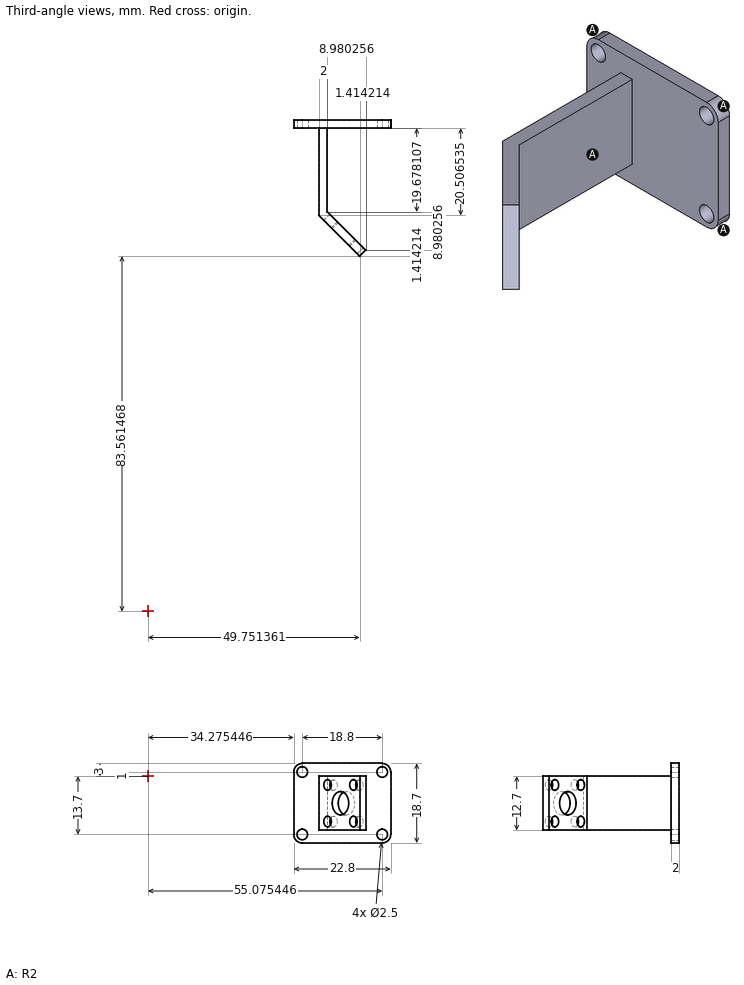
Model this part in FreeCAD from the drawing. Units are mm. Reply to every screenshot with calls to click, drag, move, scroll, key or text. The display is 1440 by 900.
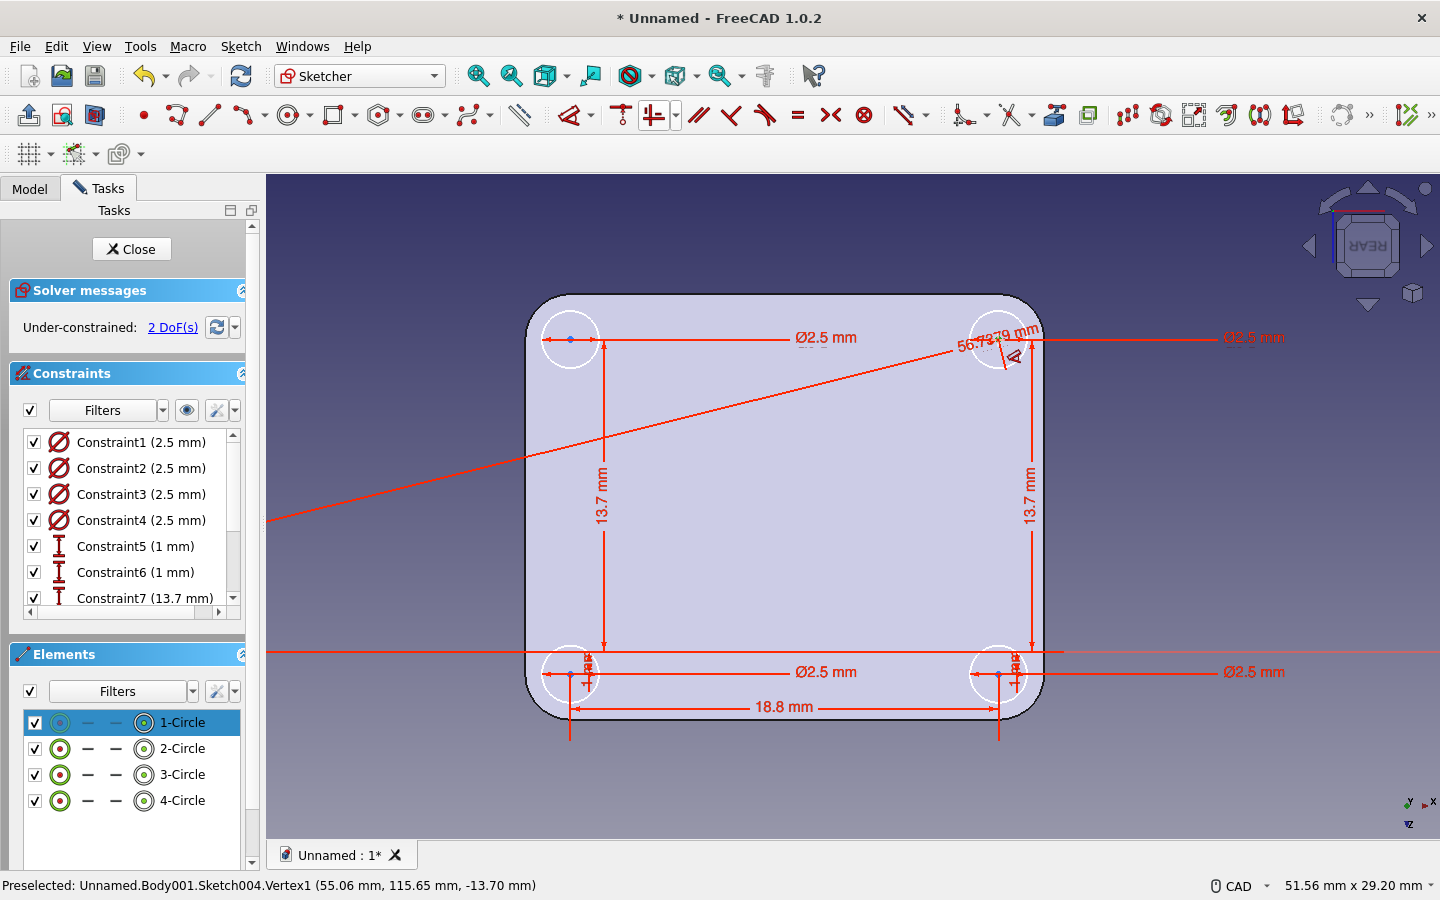
click(570, 674)
click(686, 708)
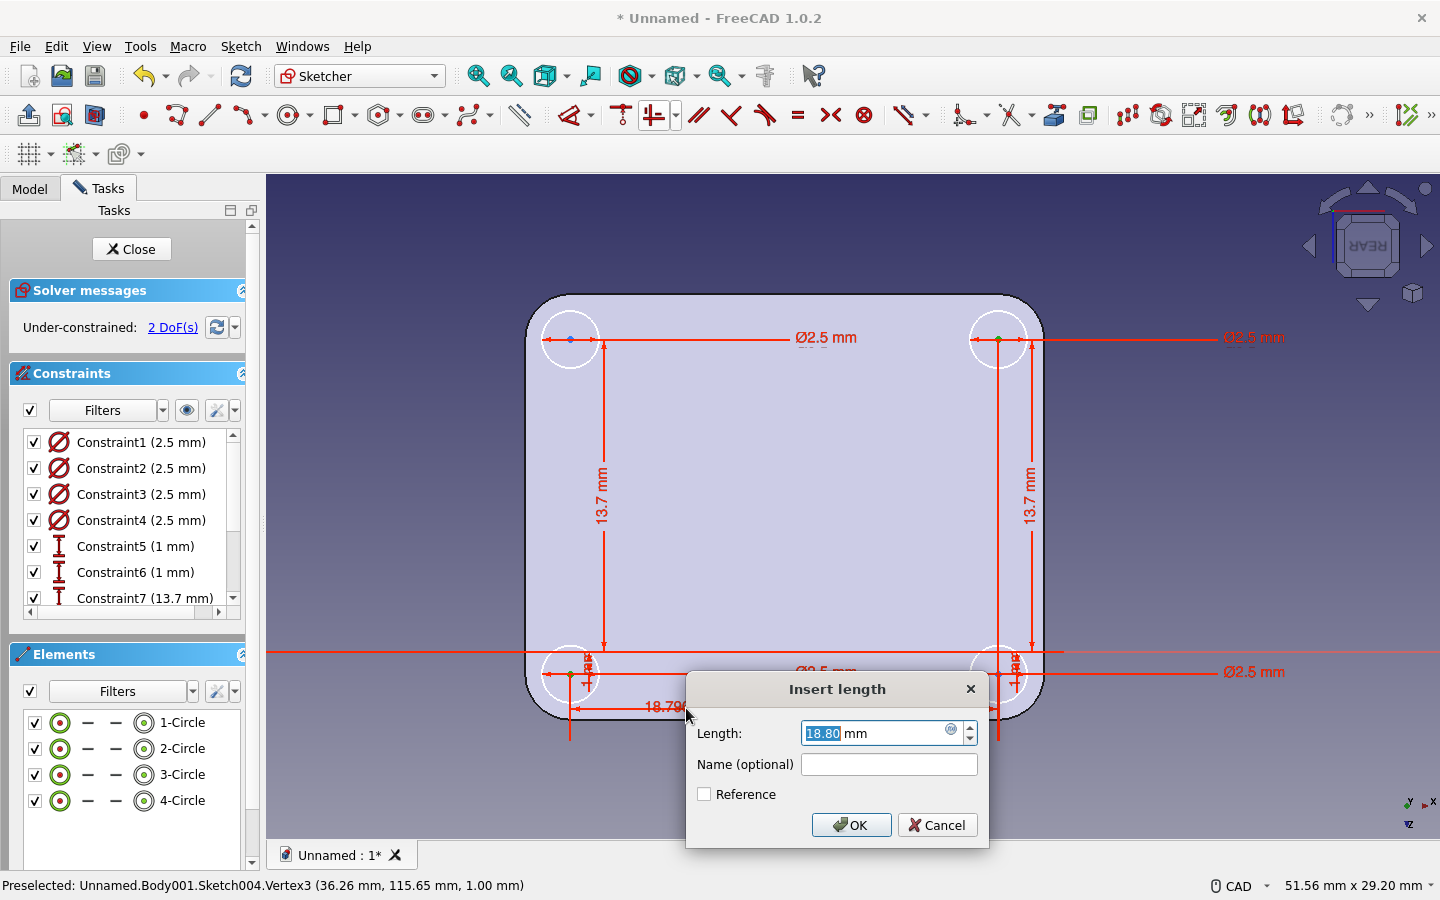
text(18.8)
key(Return)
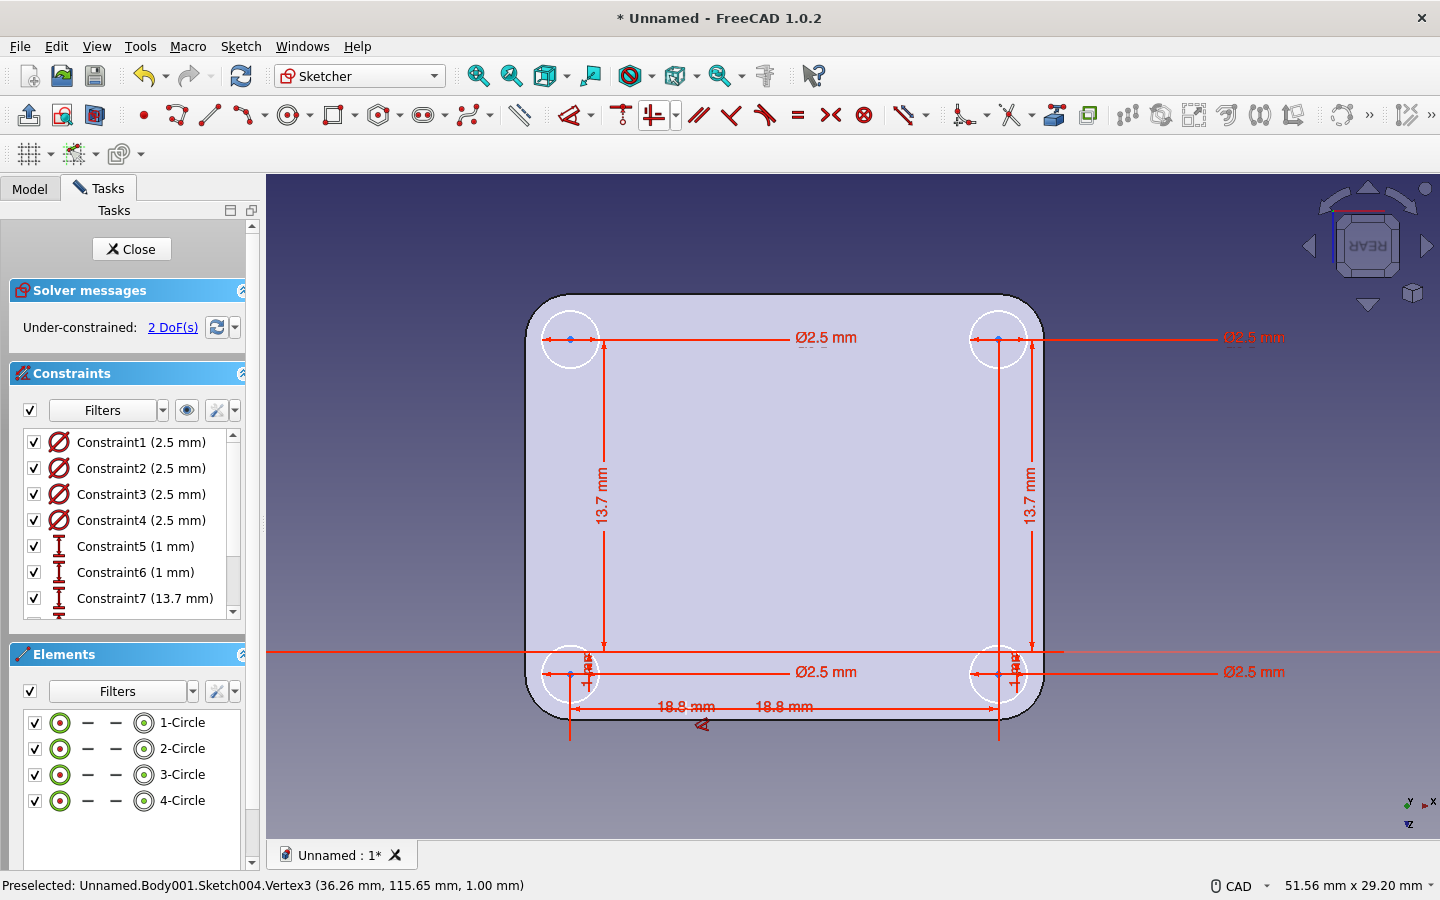
click(999, 340)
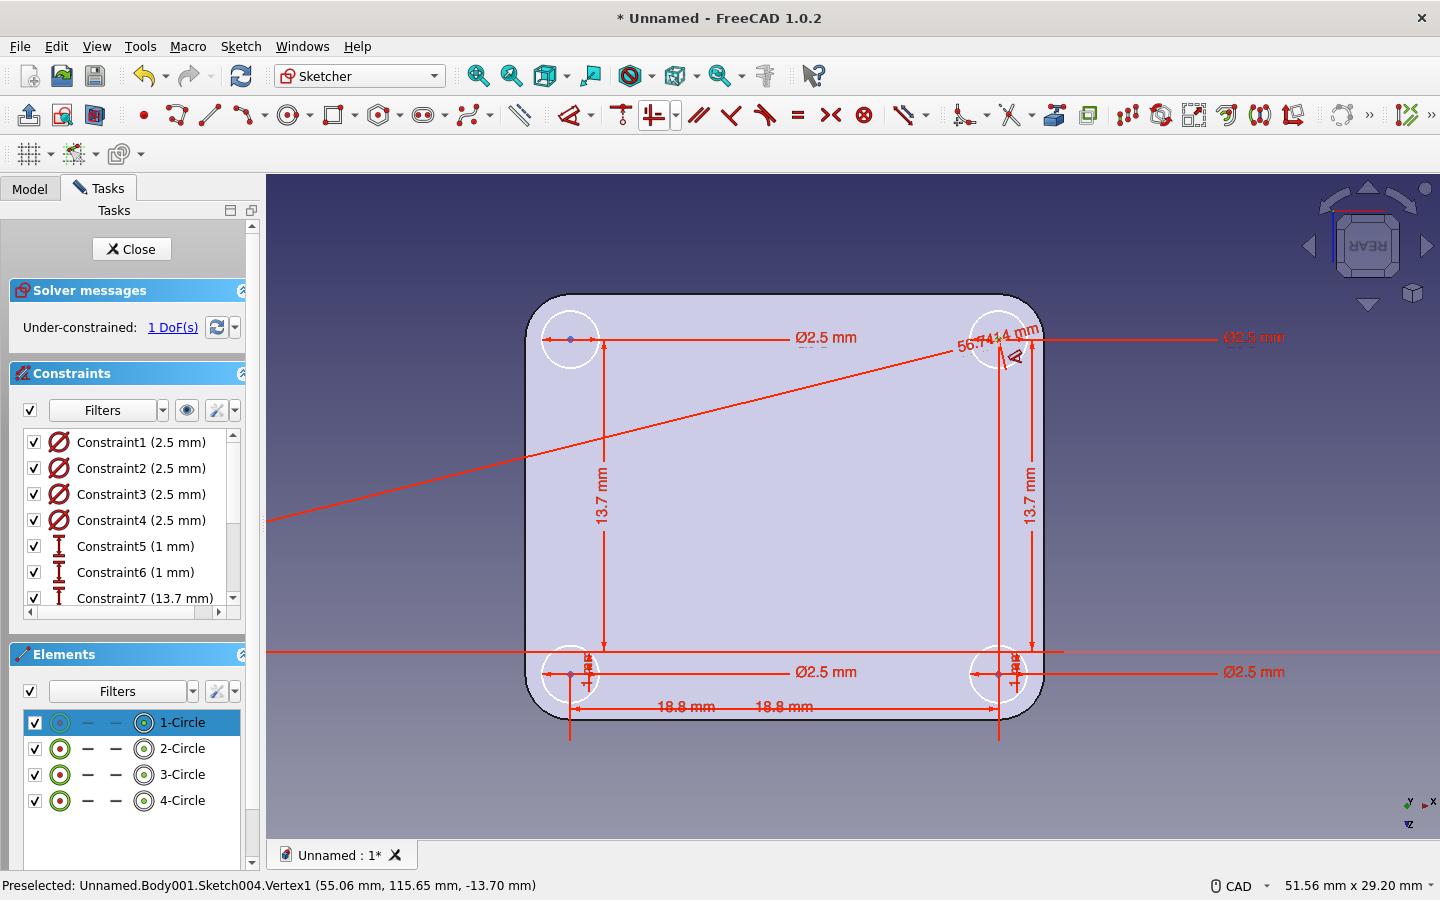
click(570, 340)
click(784, 306)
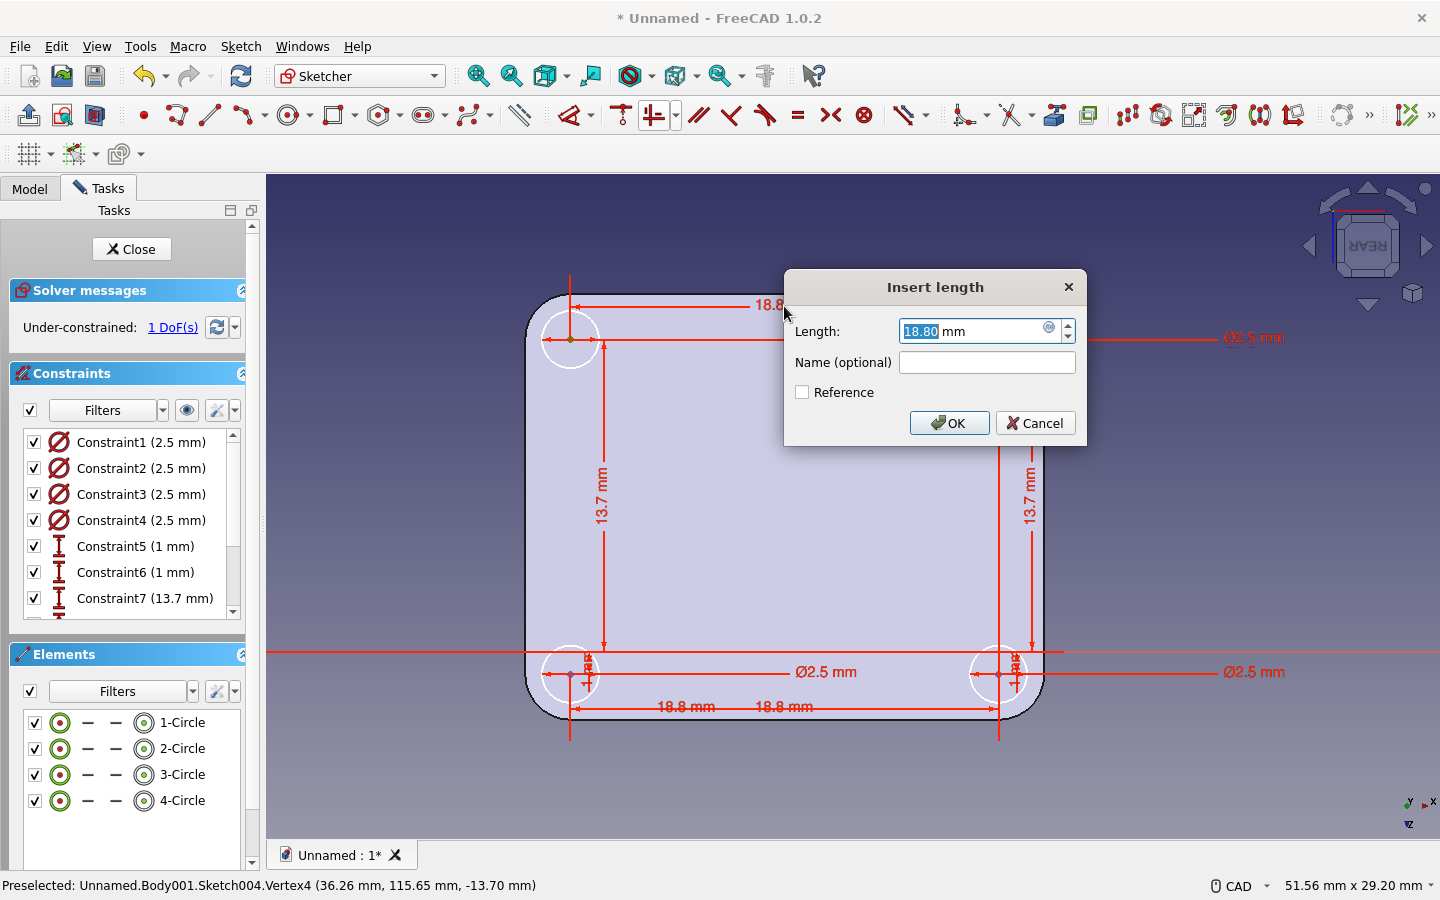
text(18.8)
key(Return)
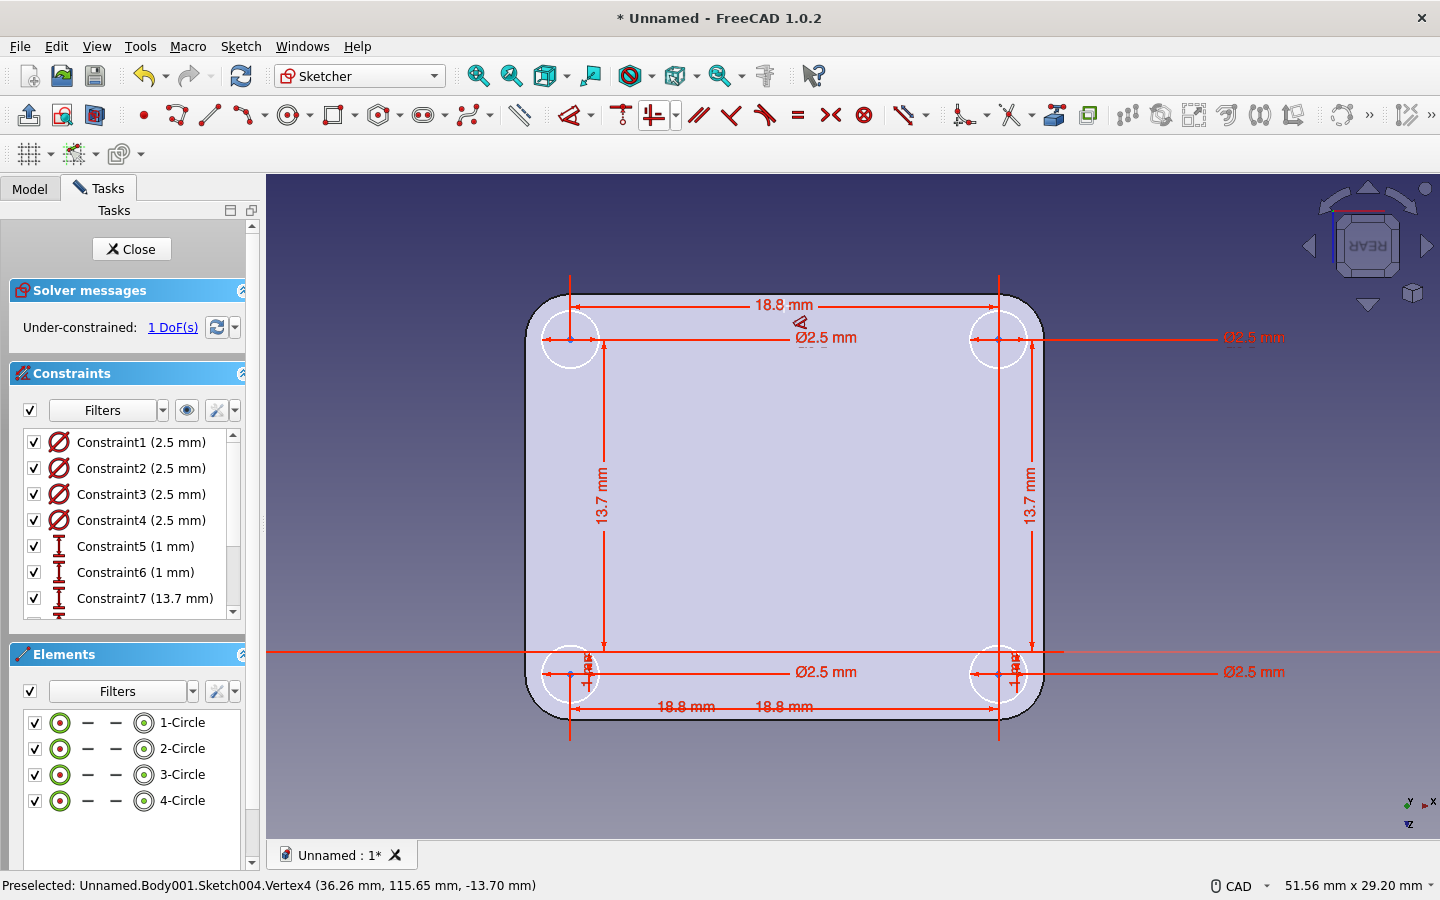
click(999, 340)
click(646, 306)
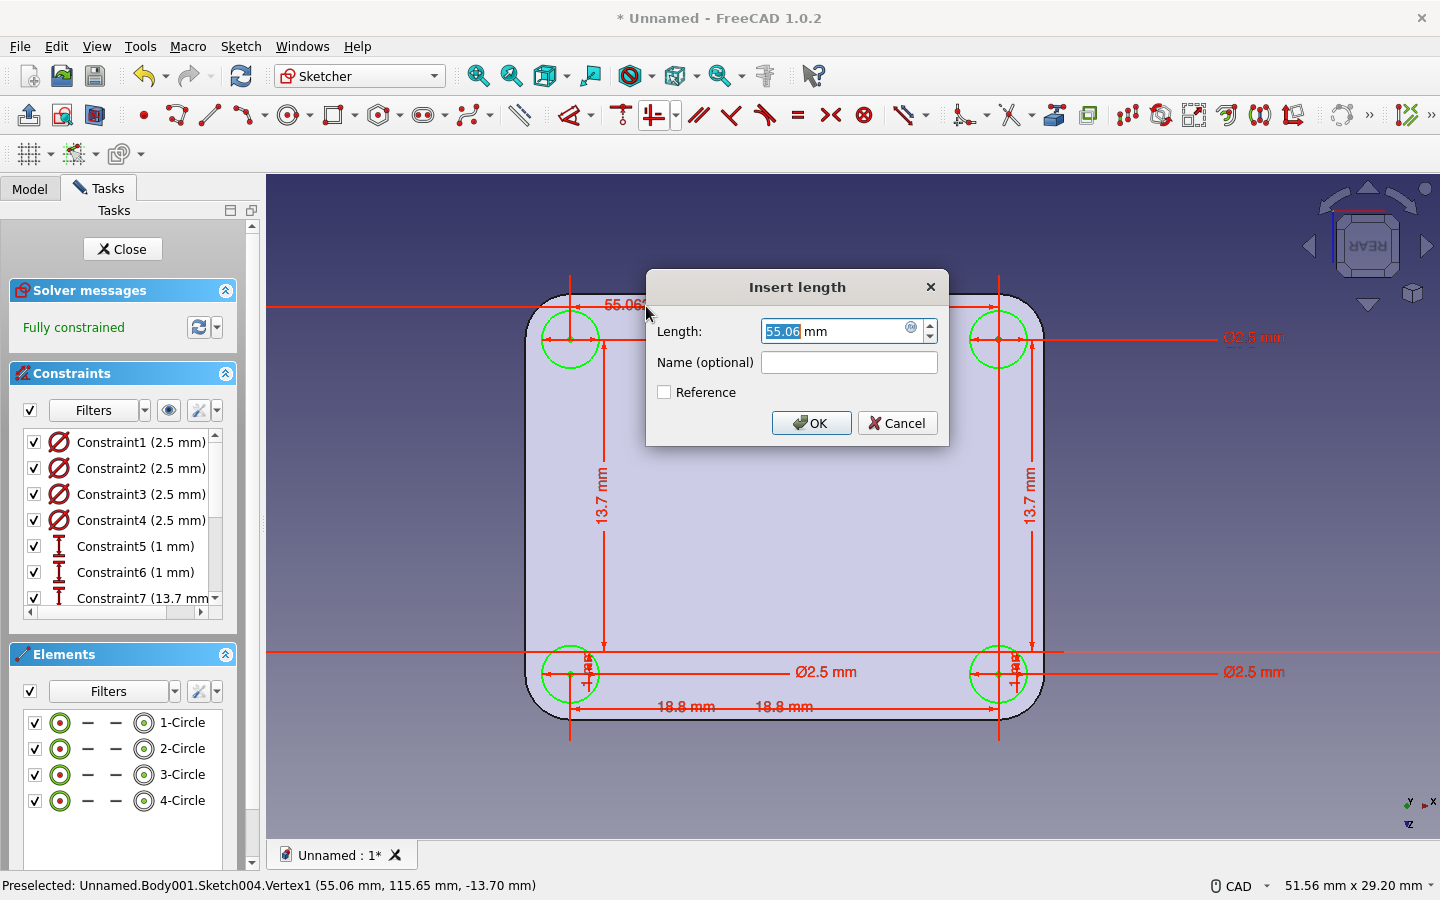
text(55.075446)
key(Return)
key(Escape)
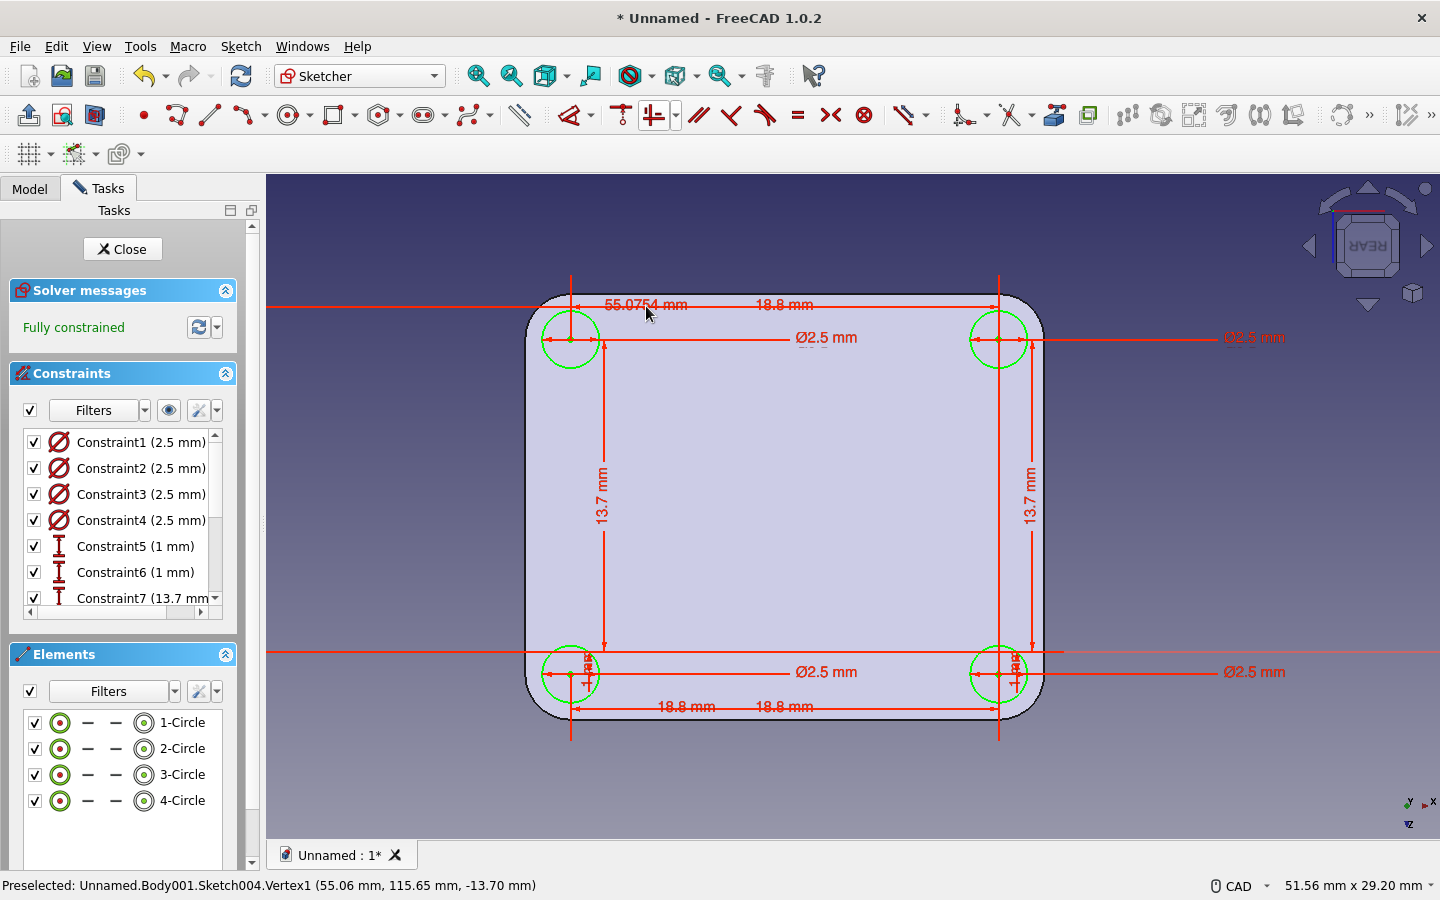
click(123, 249)